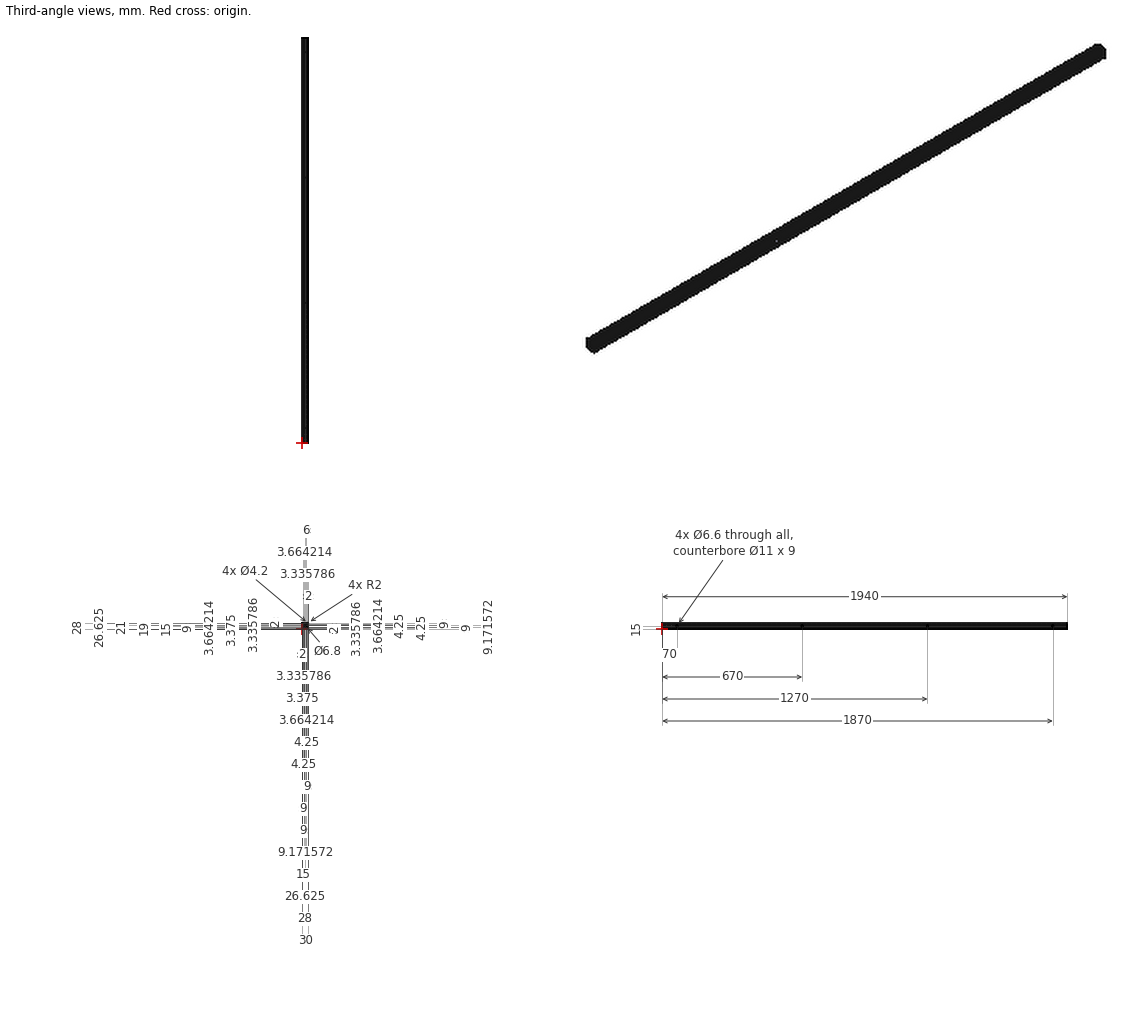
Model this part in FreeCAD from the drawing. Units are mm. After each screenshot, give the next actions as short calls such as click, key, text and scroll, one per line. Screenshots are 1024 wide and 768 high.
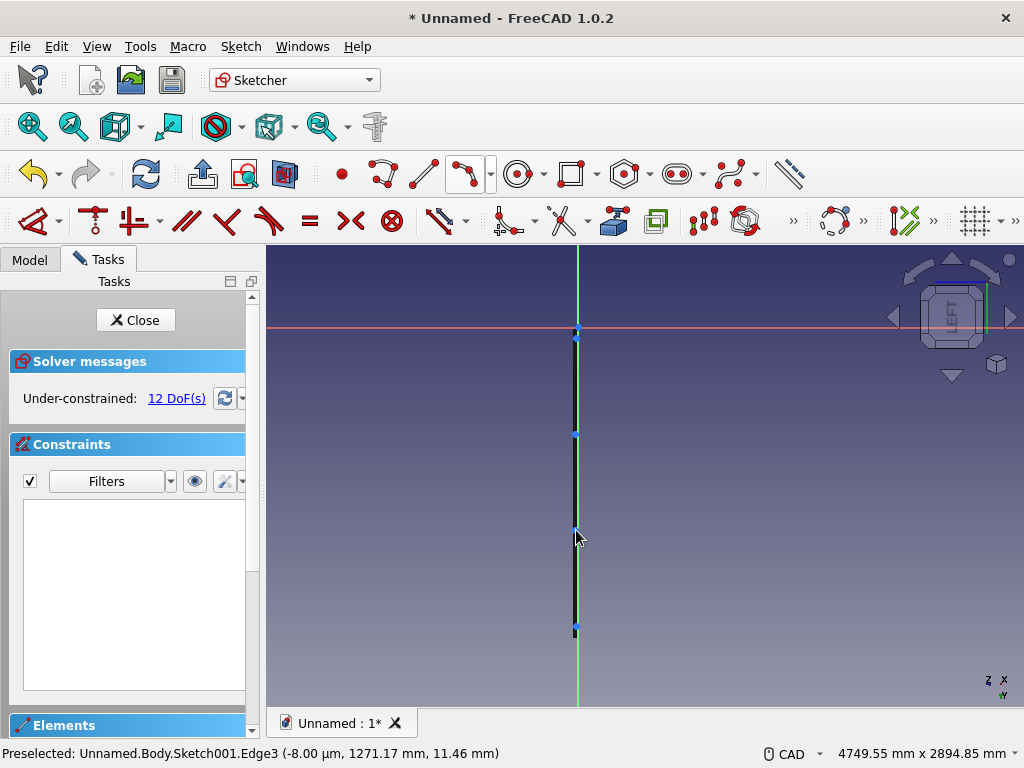
scroll(576, 434, up, 14)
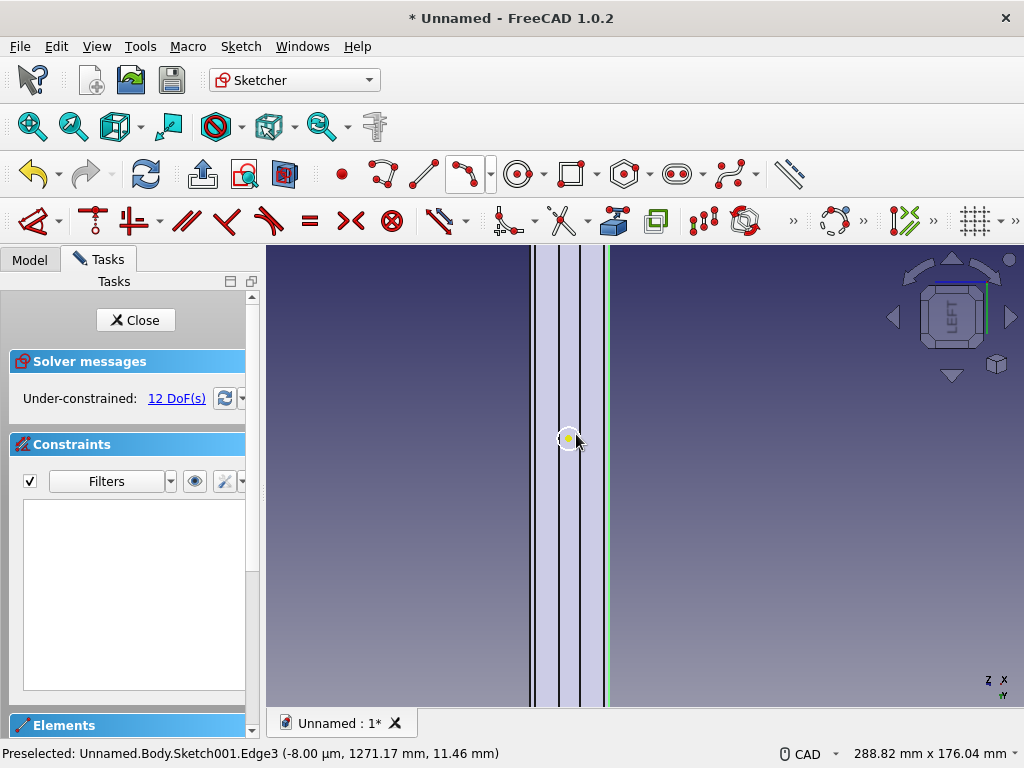
click(577, 431)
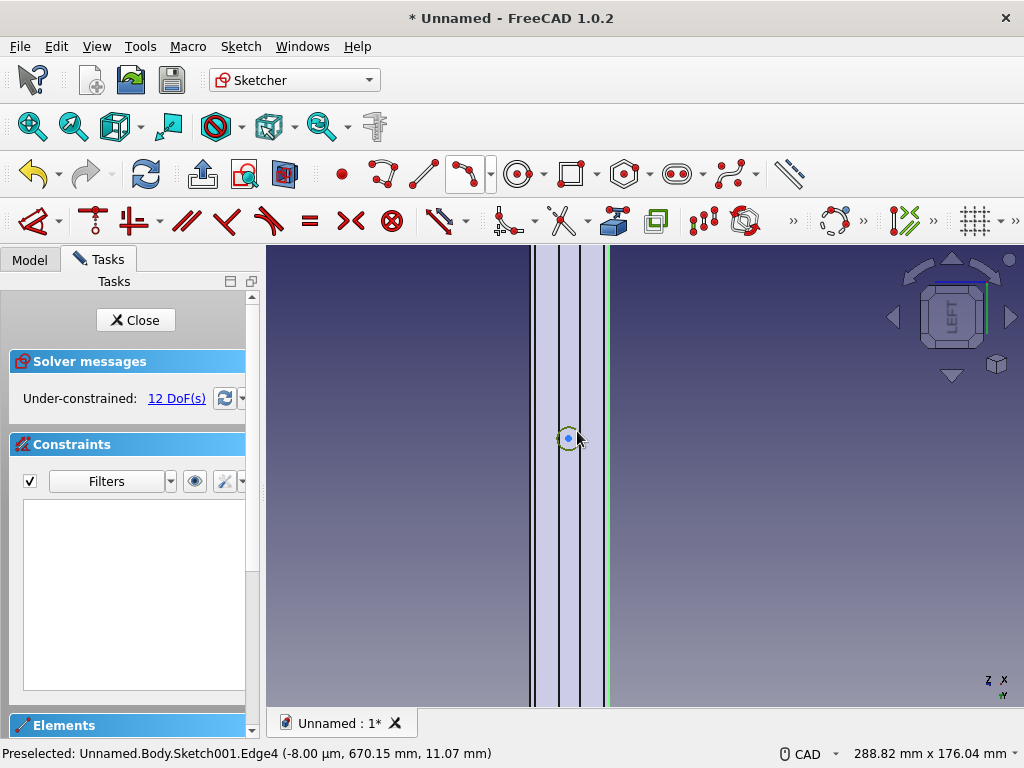
click(310, 222)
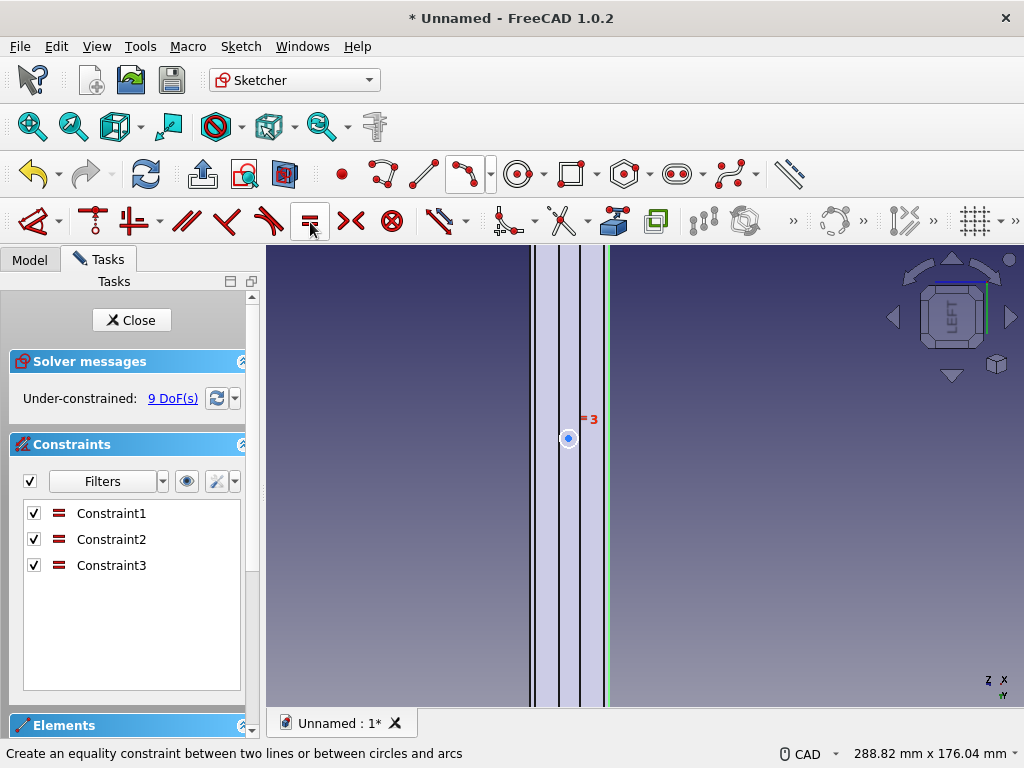
scroll(576, 433, down, 14)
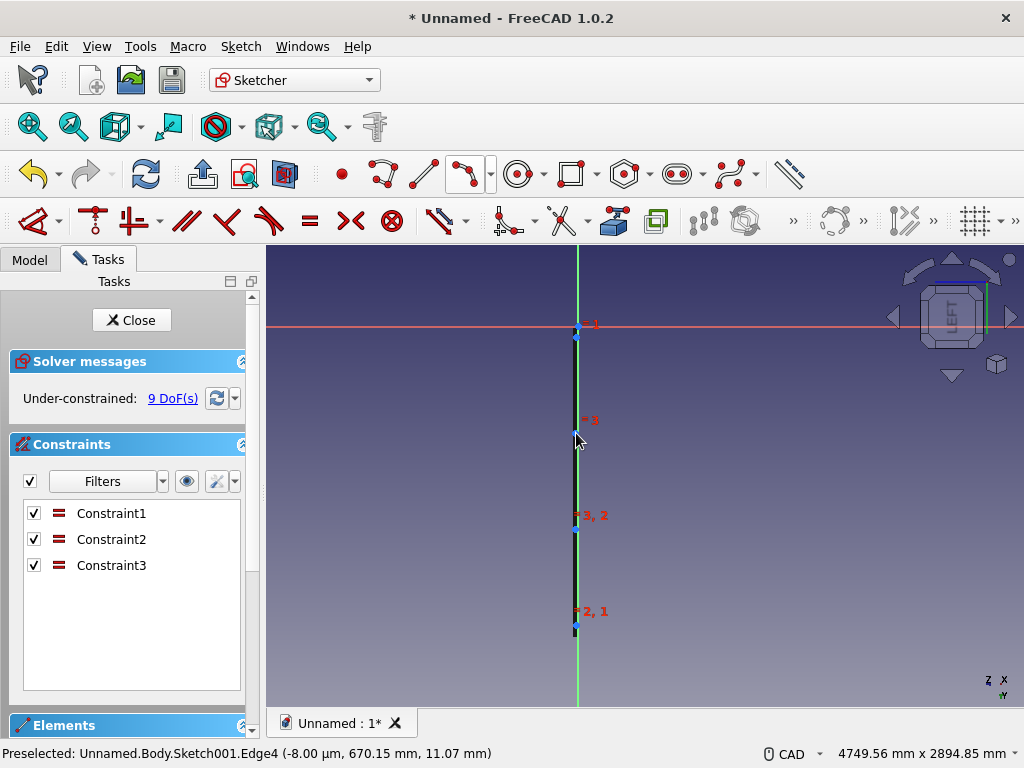
click(576, 338)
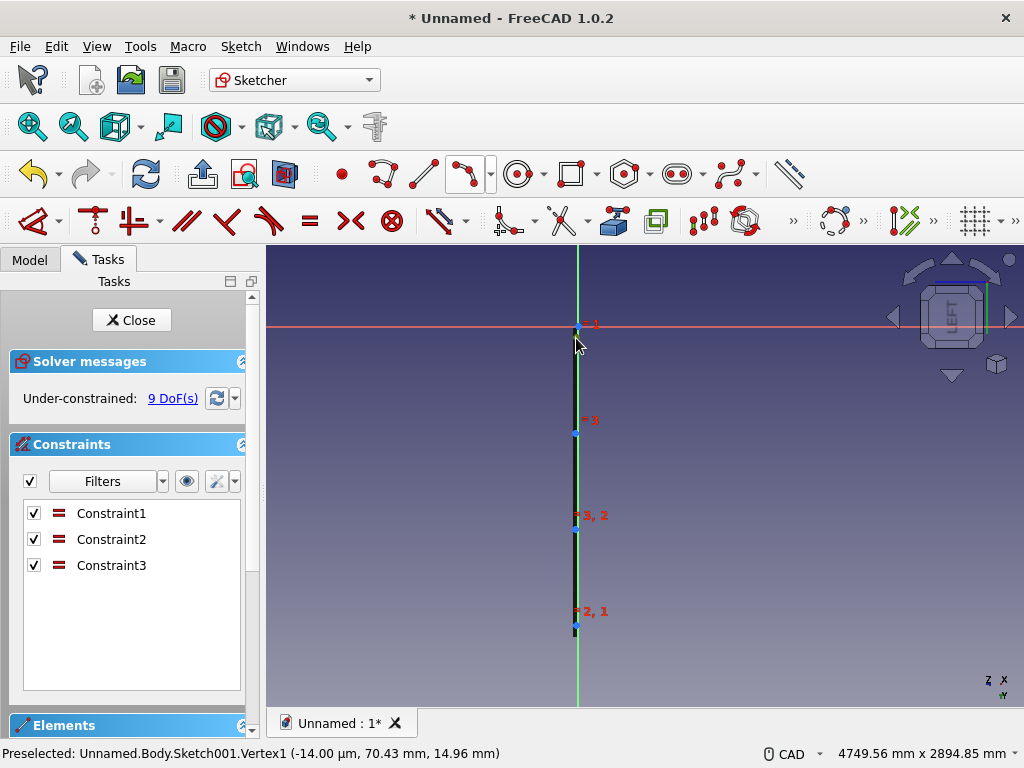
click(576, 625)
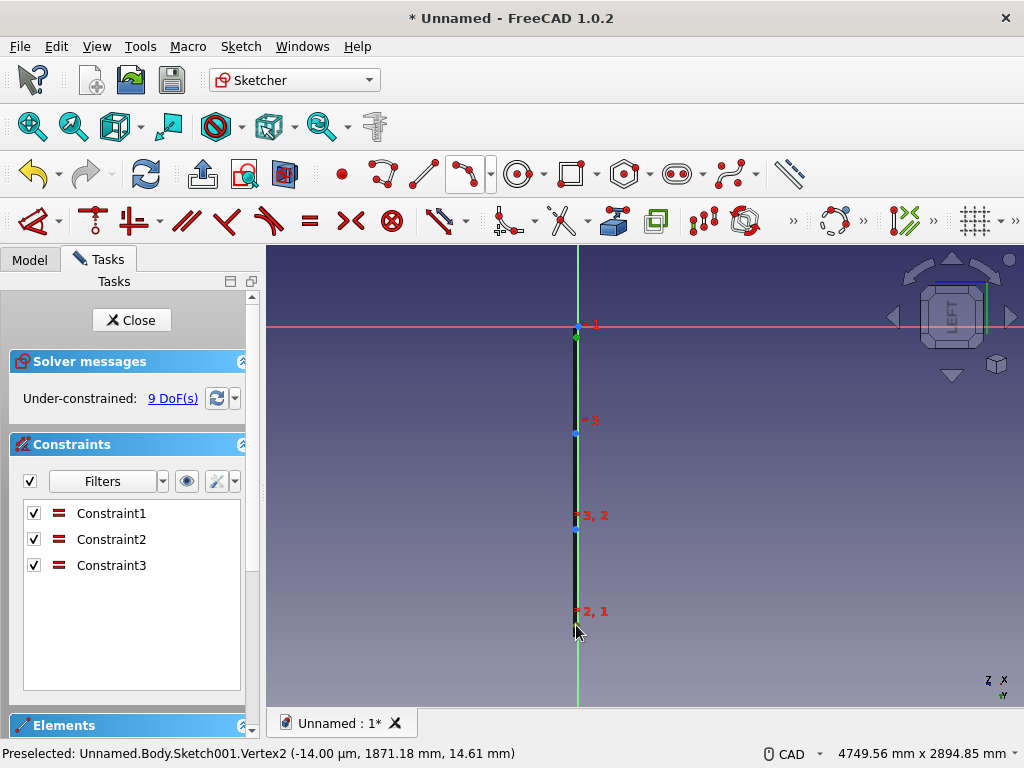
key(v)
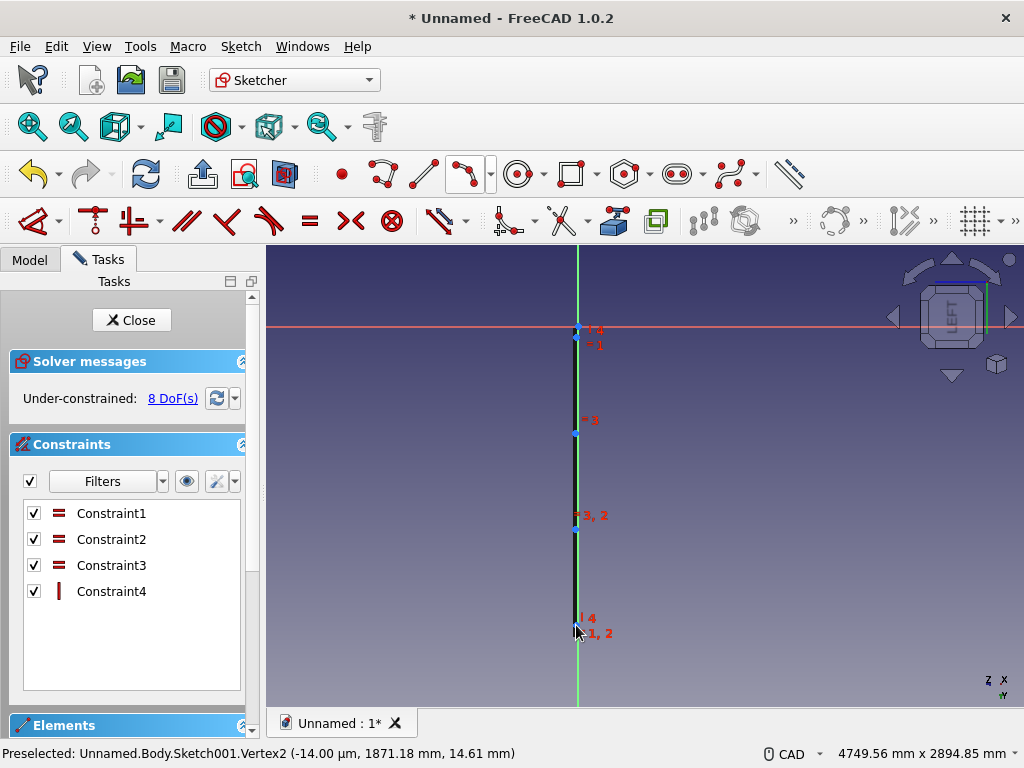
click(576, 625)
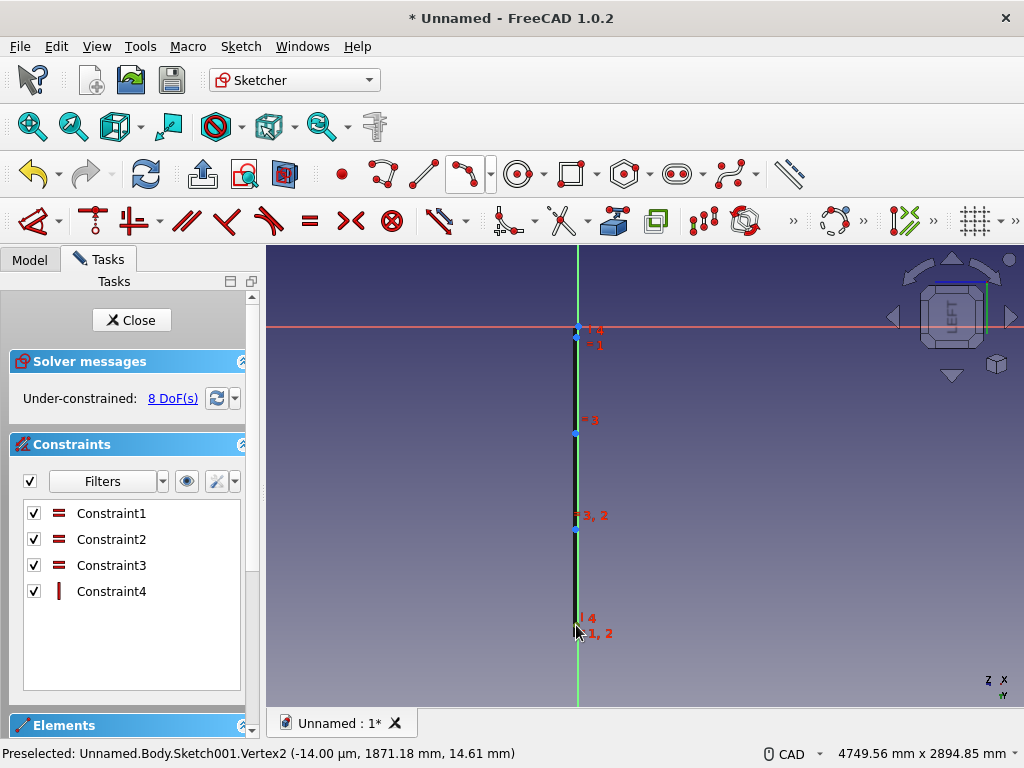
click(576, 529)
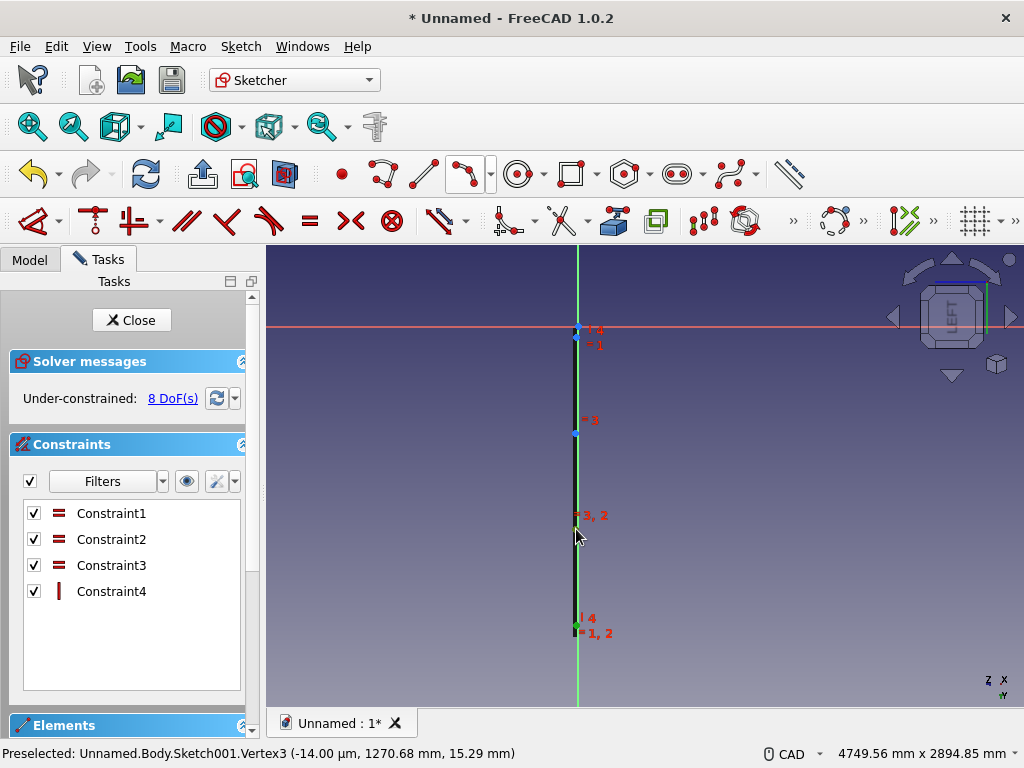
click(160, 222)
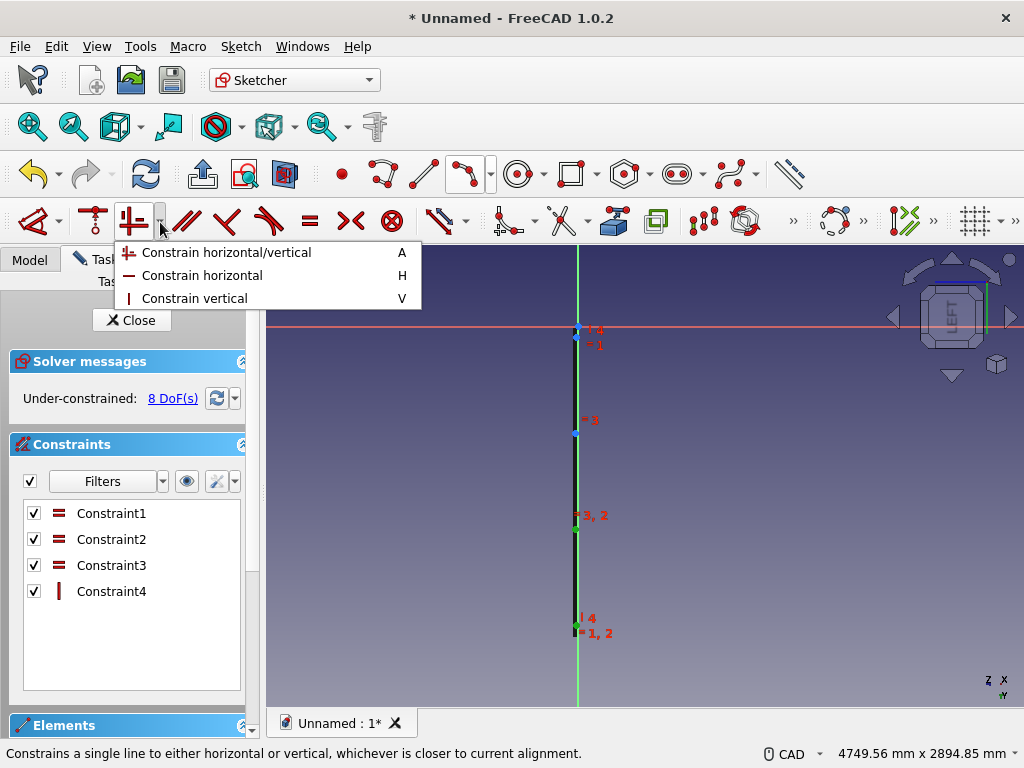
click(268, 298)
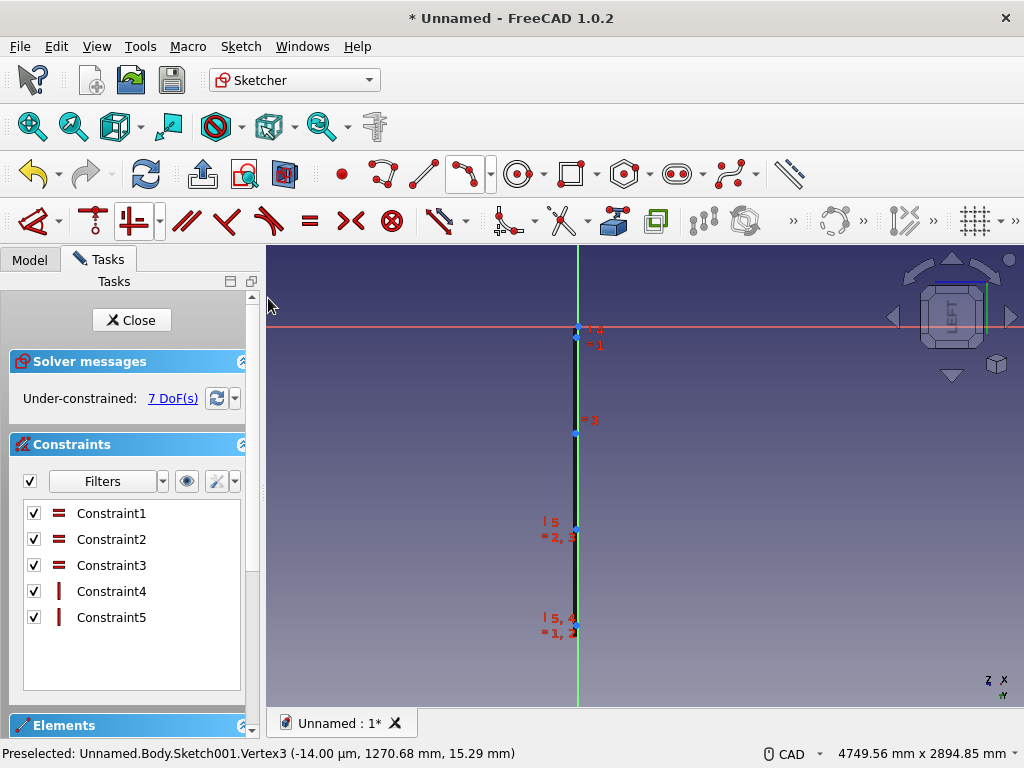
click(576, 338)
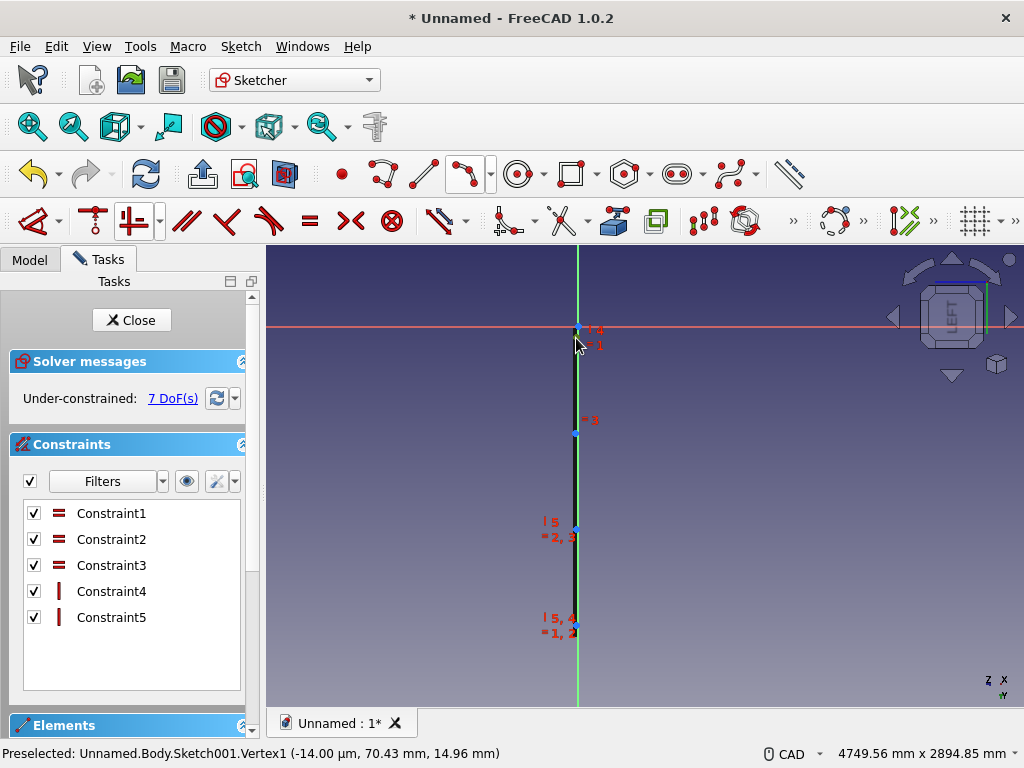
click(576, 434)